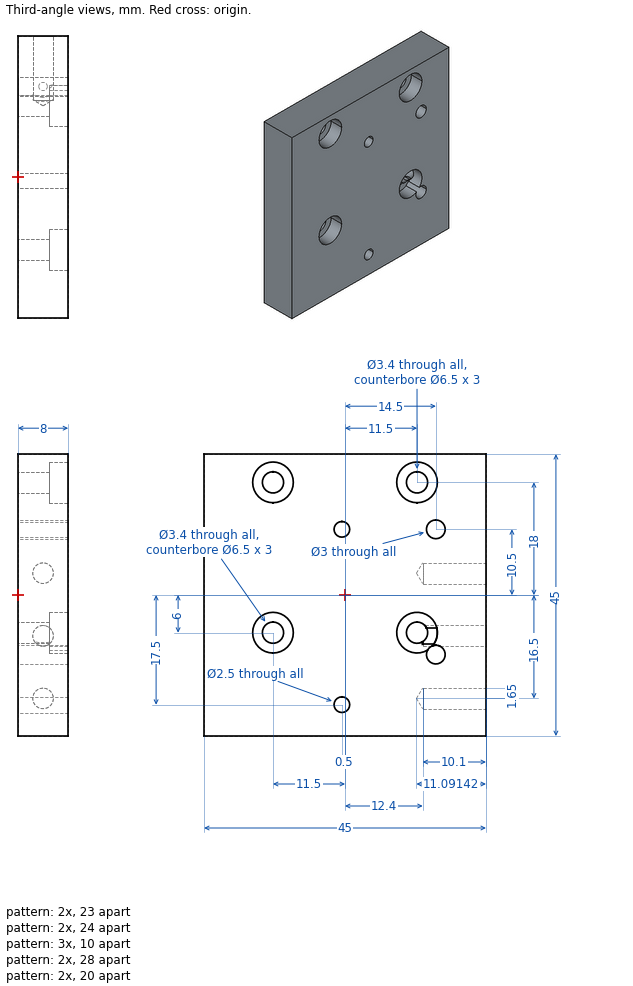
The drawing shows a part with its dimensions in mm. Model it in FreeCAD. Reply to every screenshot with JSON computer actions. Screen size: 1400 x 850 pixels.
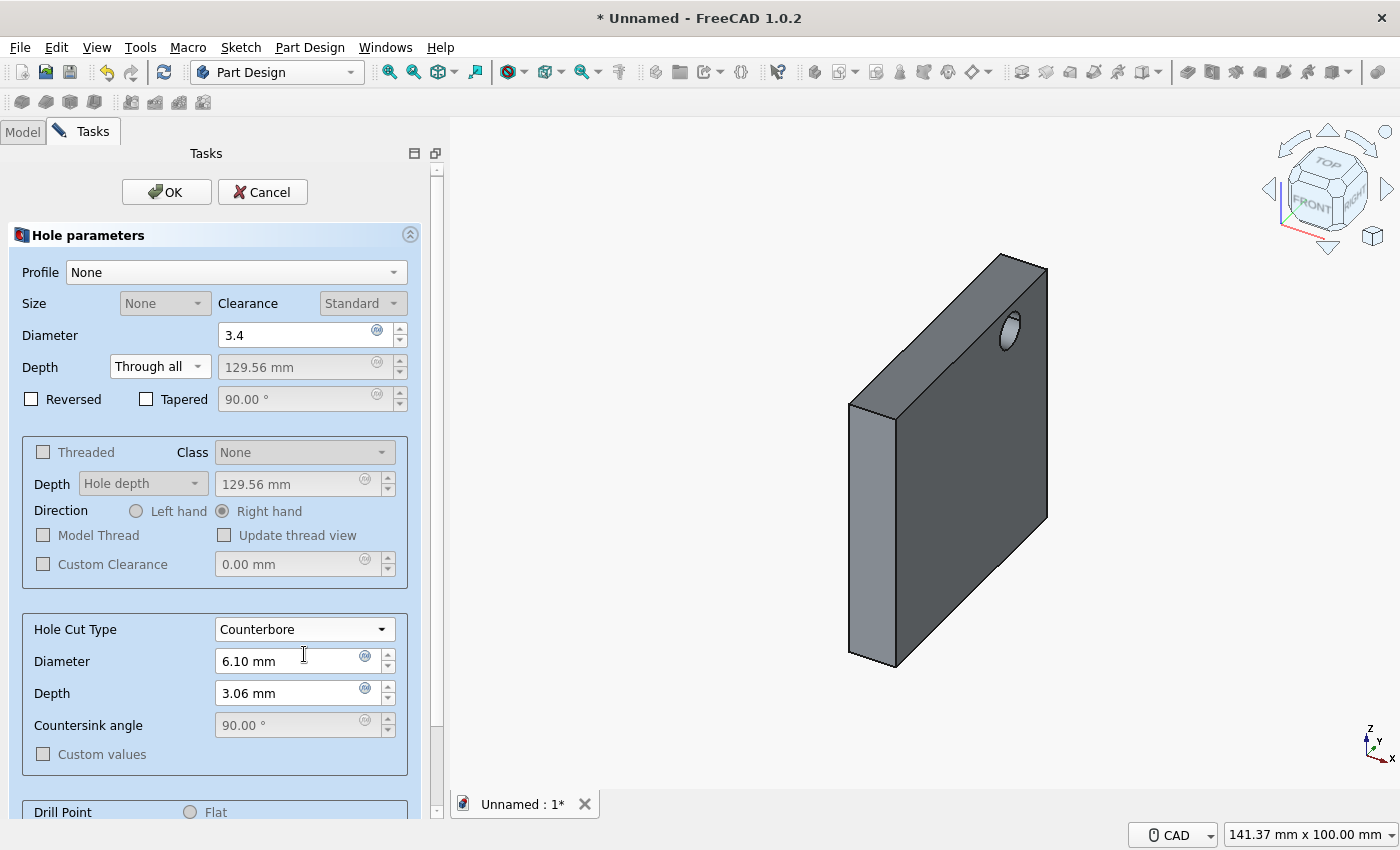
{"action": "triple_click", "coordinate": [298, 661]}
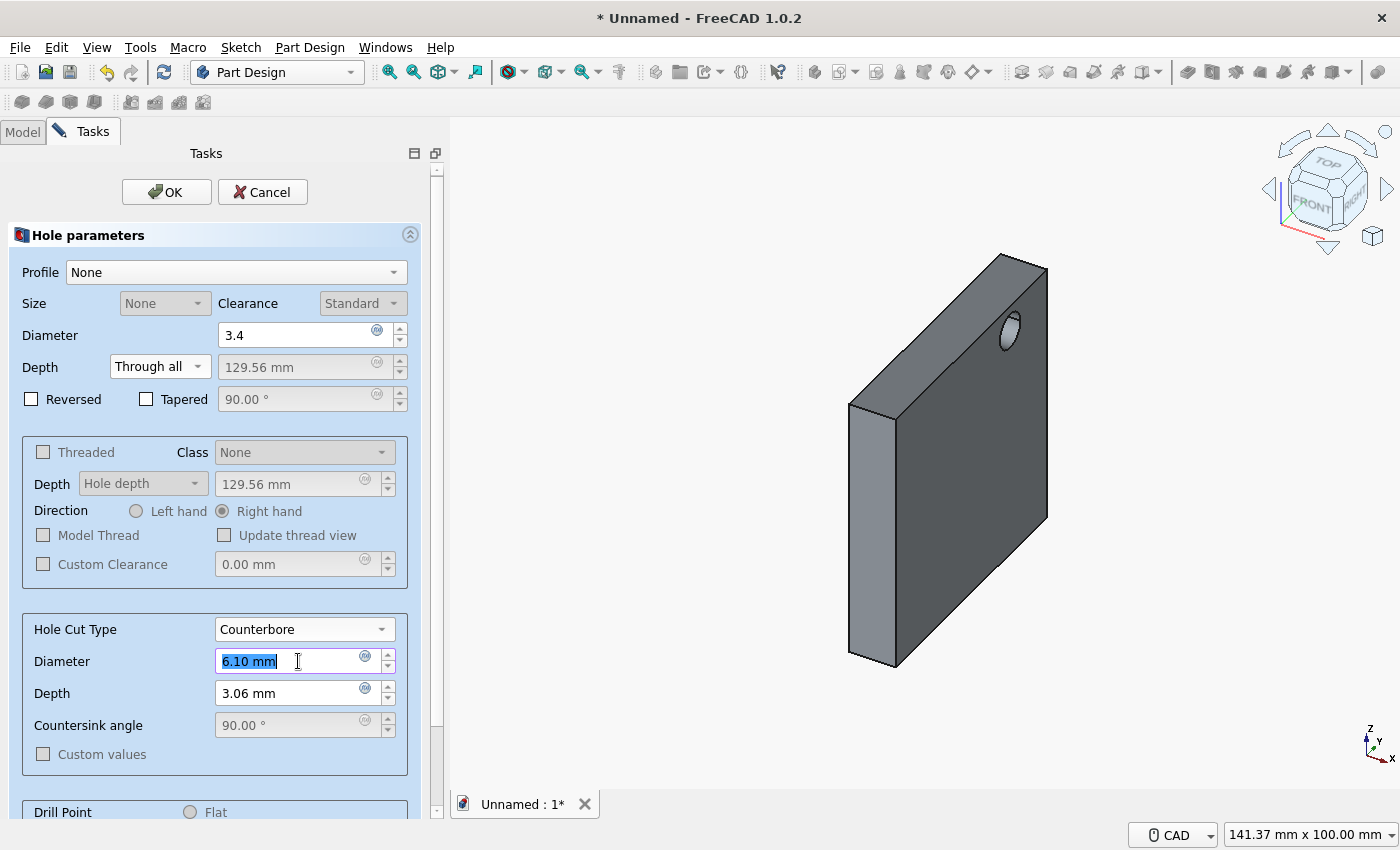
{"action": "type", "text": "6.5"}
{"action": "key", "text": "Tab"}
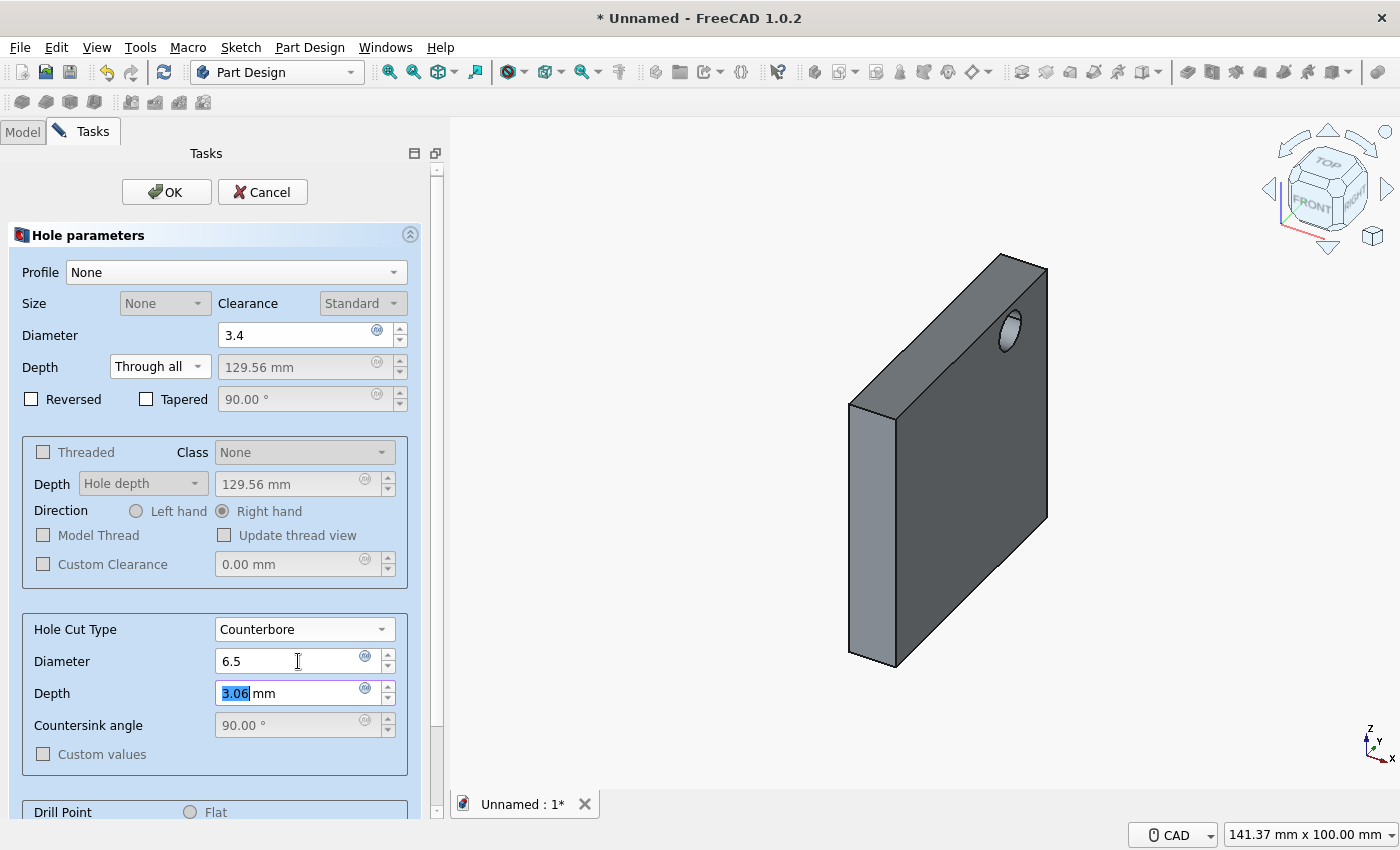
{"action": "type", "text": "3"}
{"action": "key", "text": "Tab"}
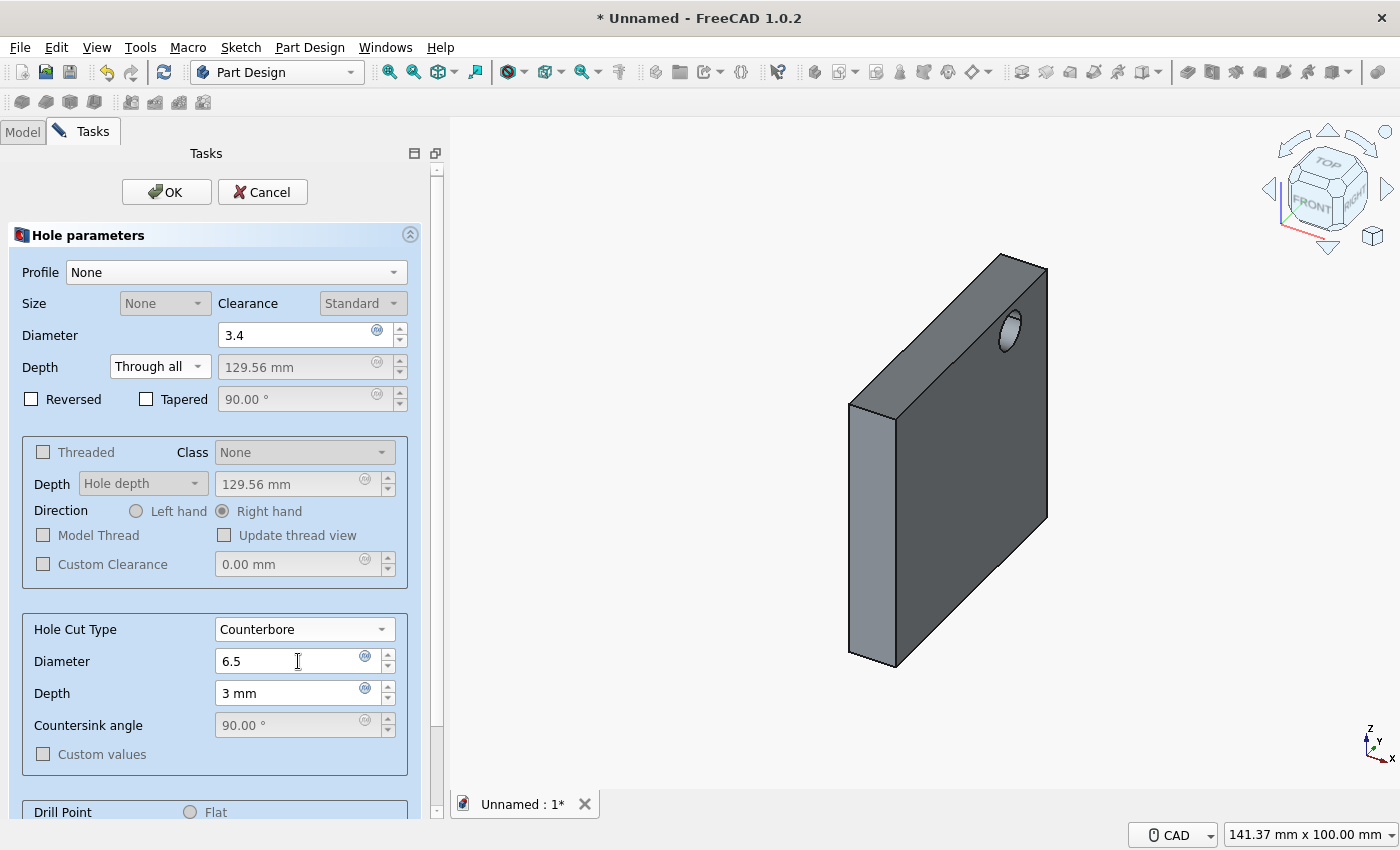
{"action": "left_click", "coordinate": [167, 192]}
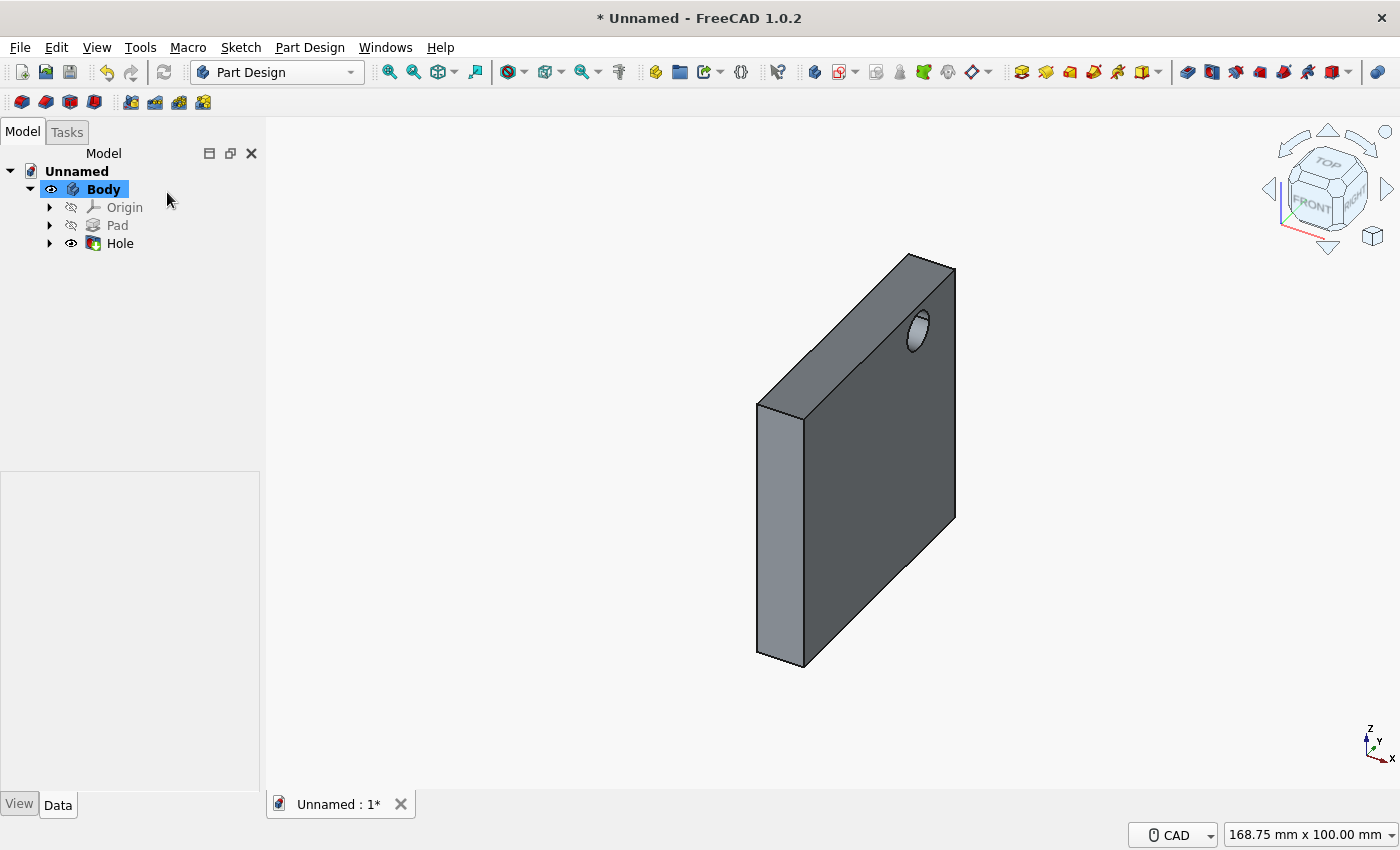
{"action": "left_click", "coordinate": [116, 243]}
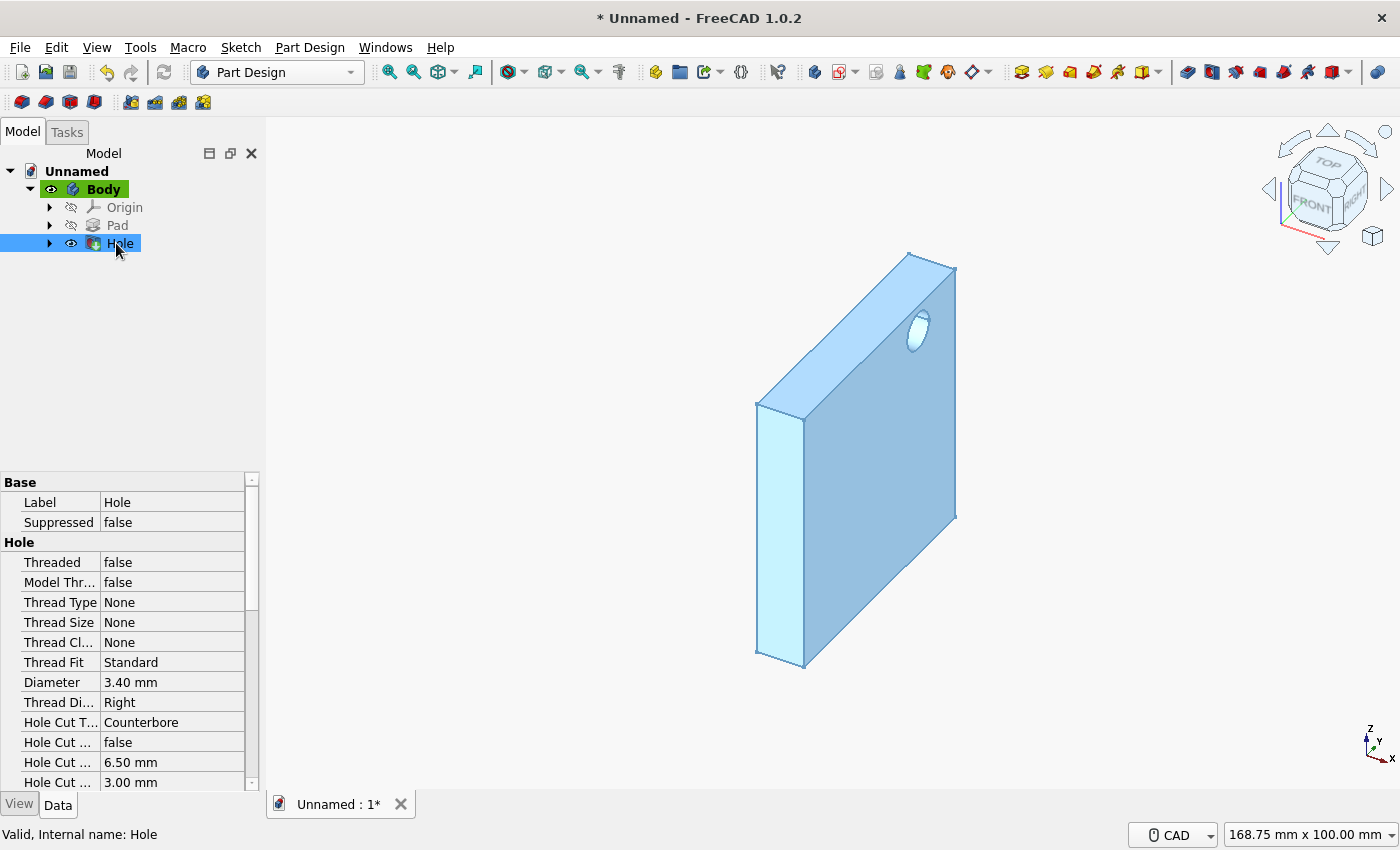
{"action": "left_click", "coordinate": [156, 102]}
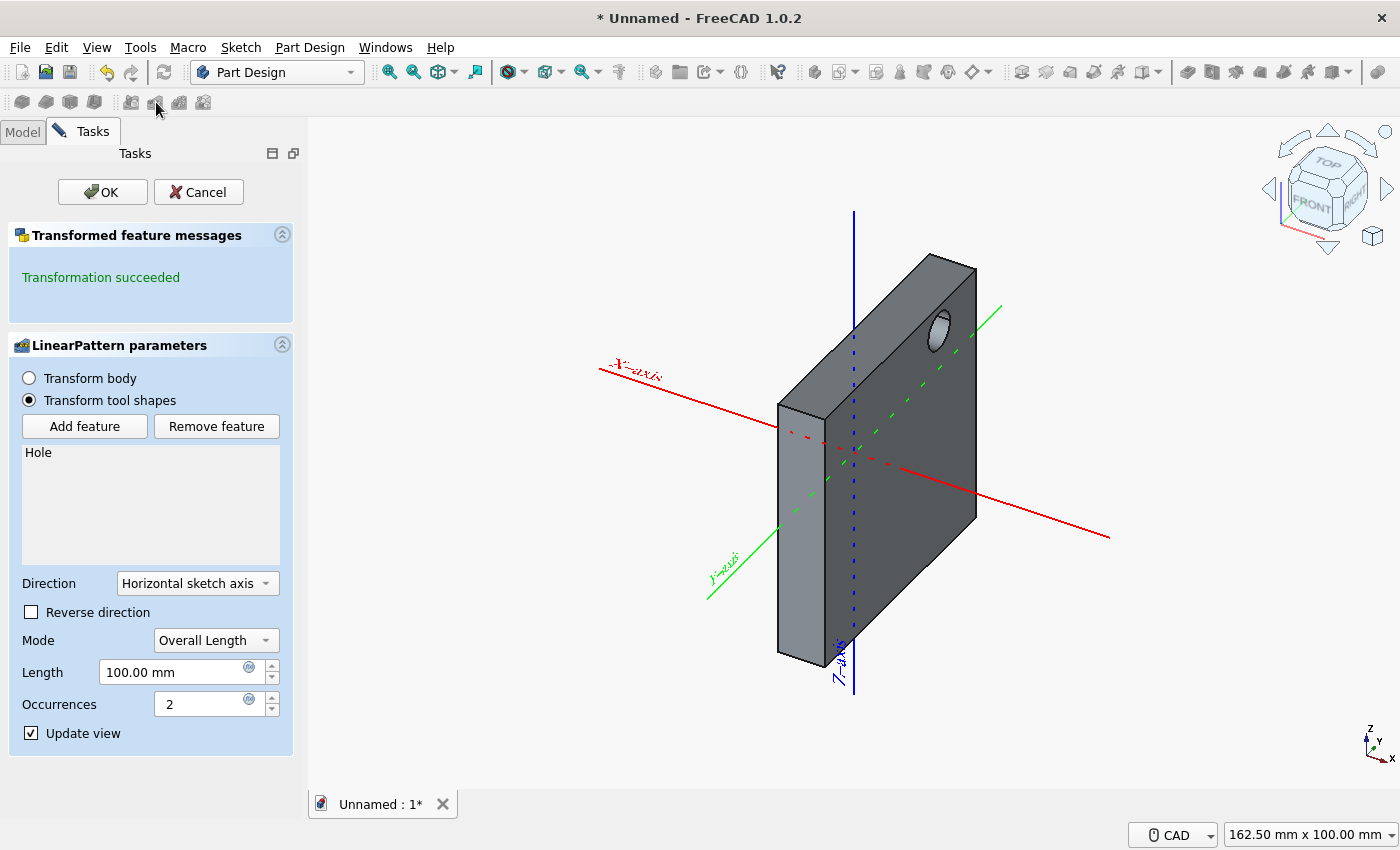
{"action": "left_click", "coordinate": [198, 584]}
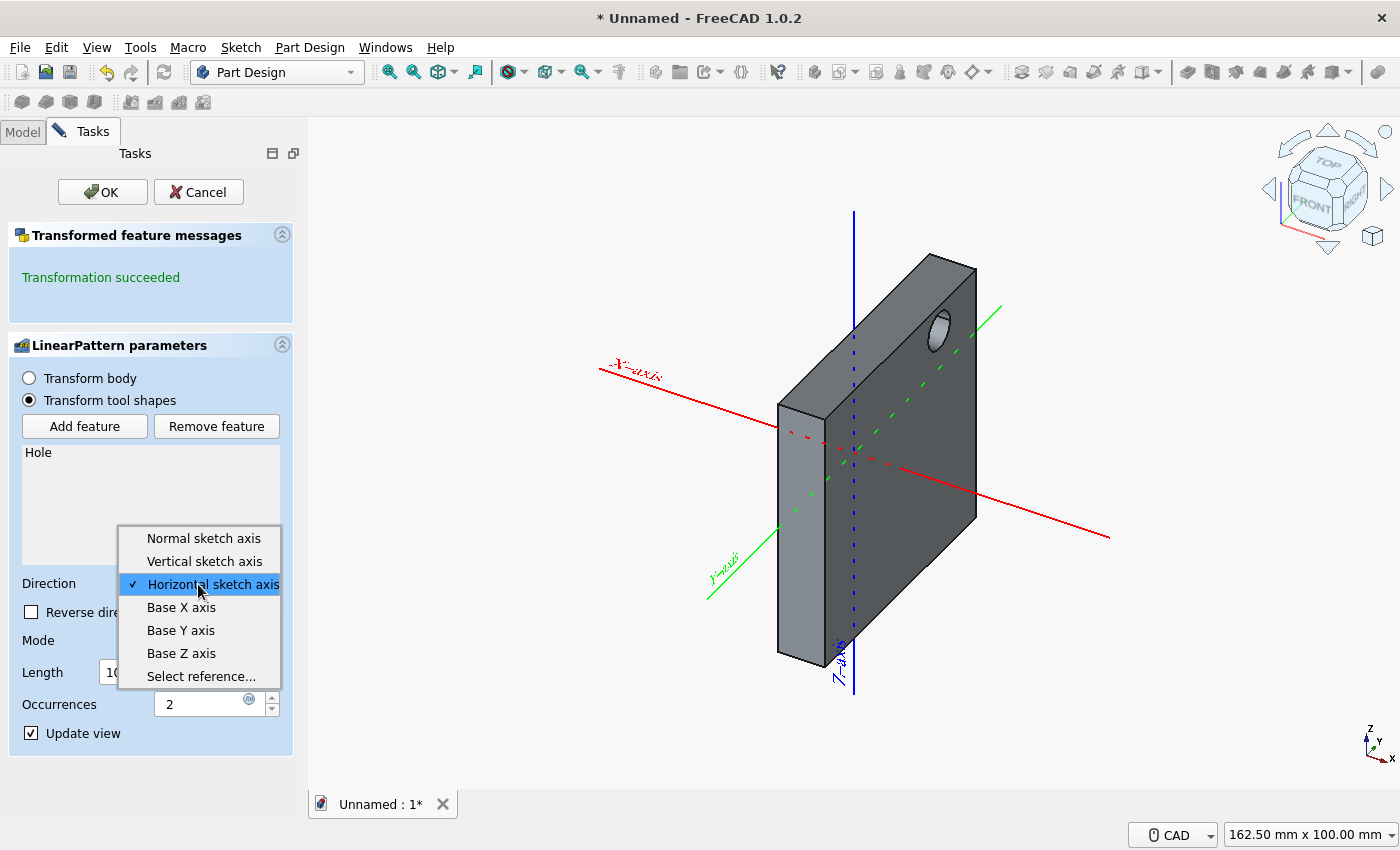
{"action": "left_click", "coordinate": [198, 630]}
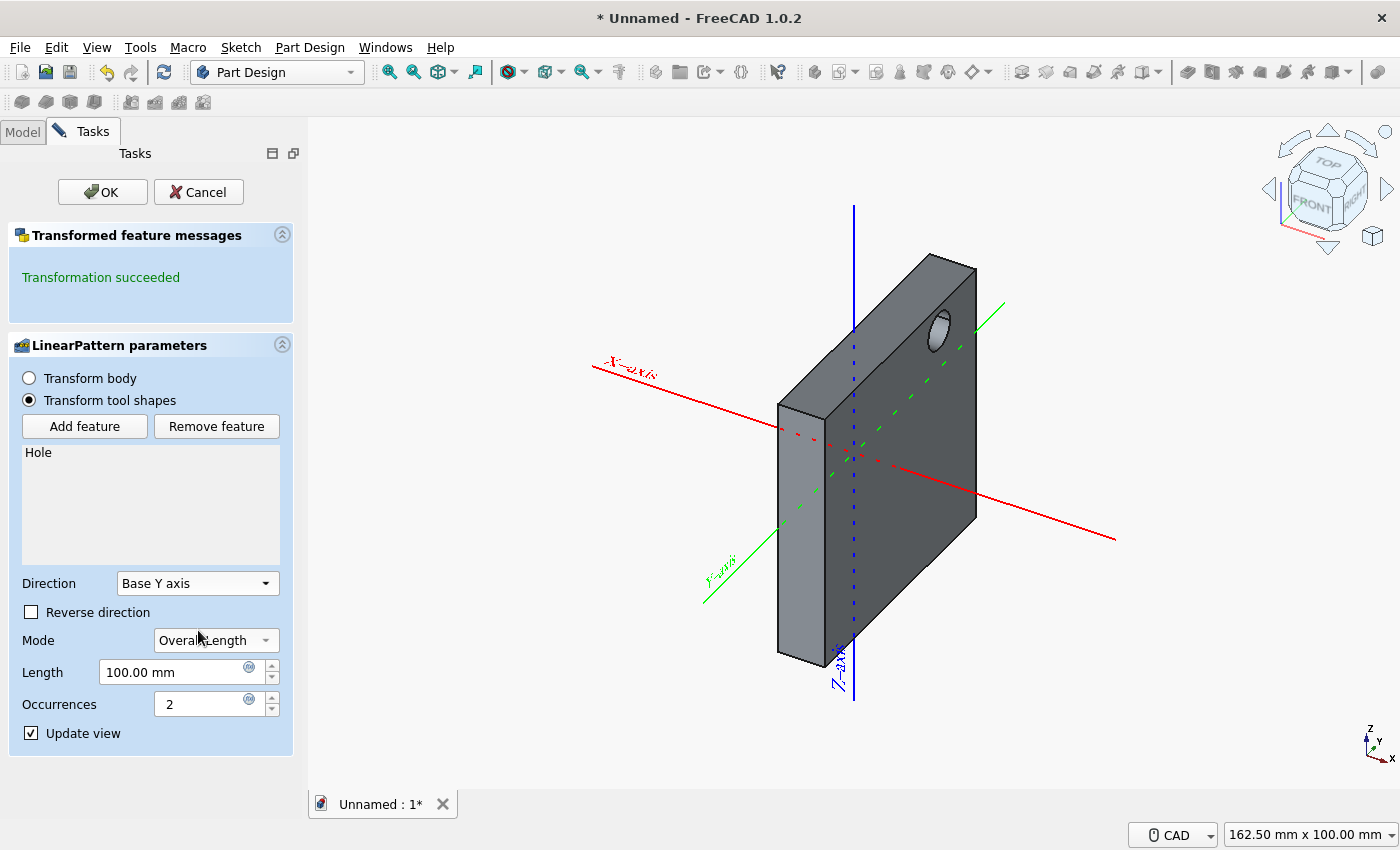
{"action": "left_click", "coordinate": [217, 640]}